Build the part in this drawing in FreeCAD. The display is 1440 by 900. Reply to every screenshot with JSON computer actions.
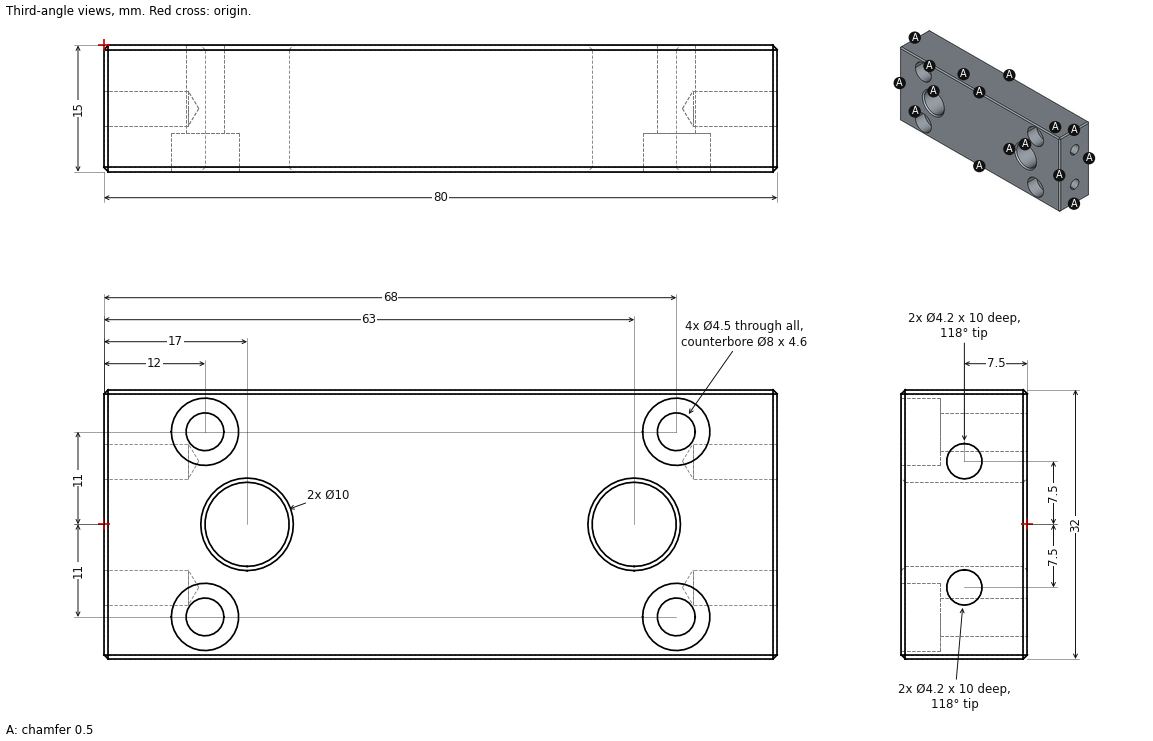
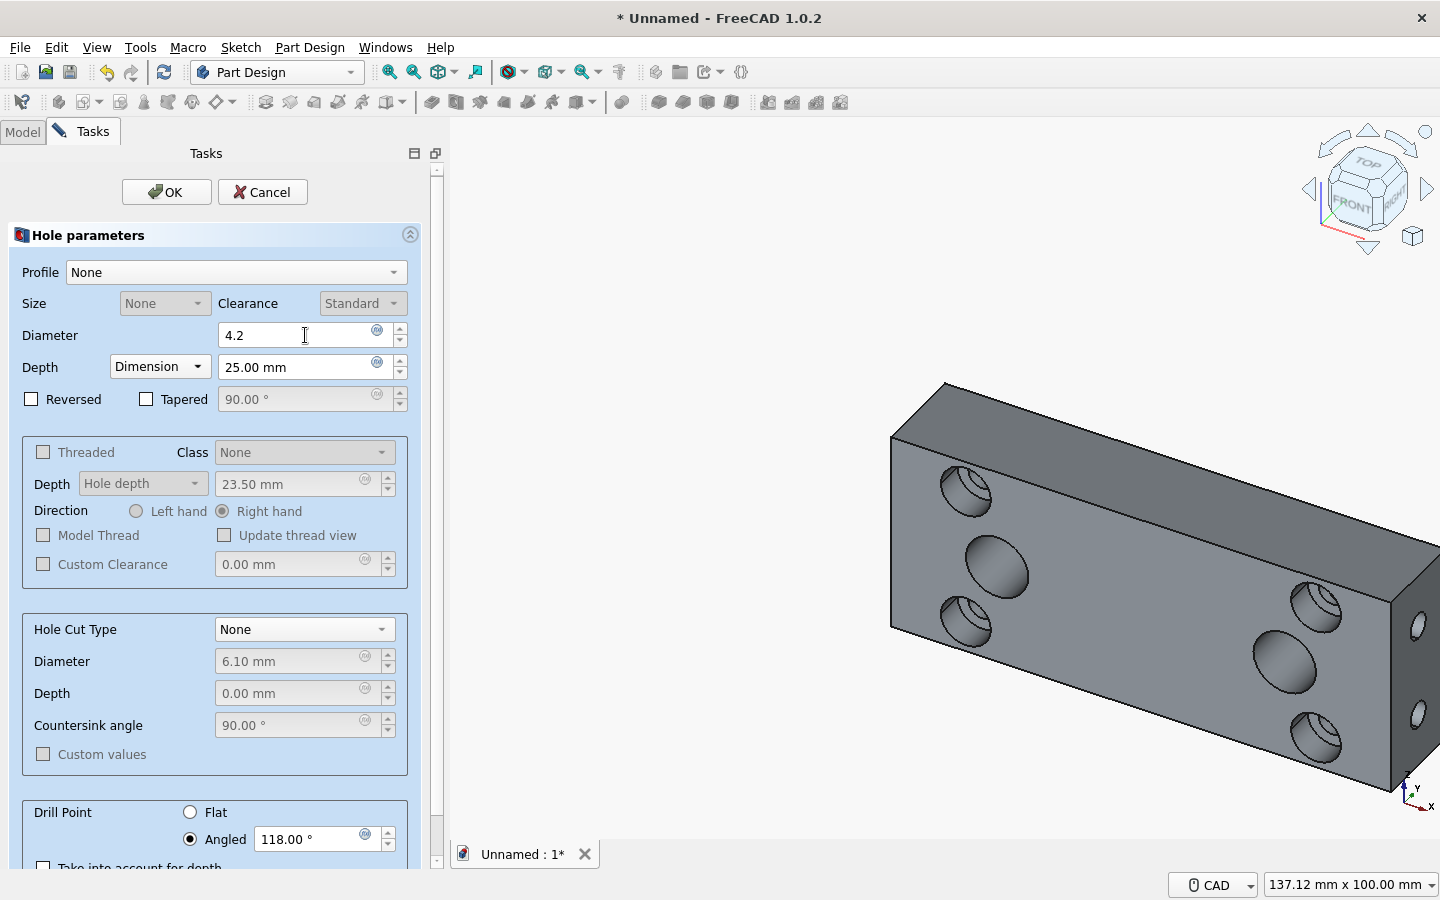
{"action": "triple_click", "coordinate": [305, 367]}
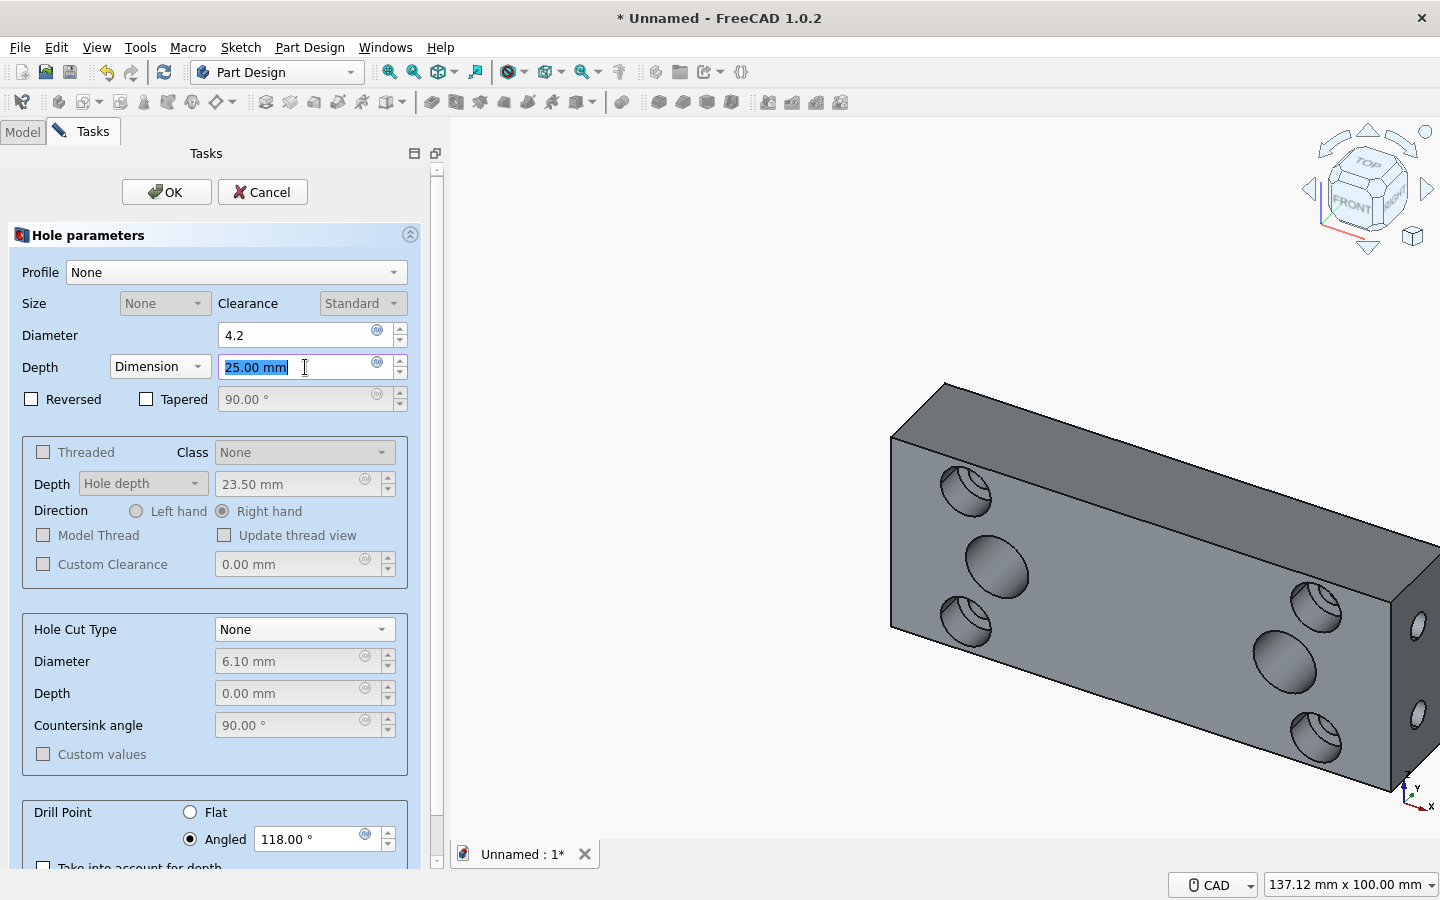
{"action": "type", "text": "10"}
{"action": "key", "text": "Tab"}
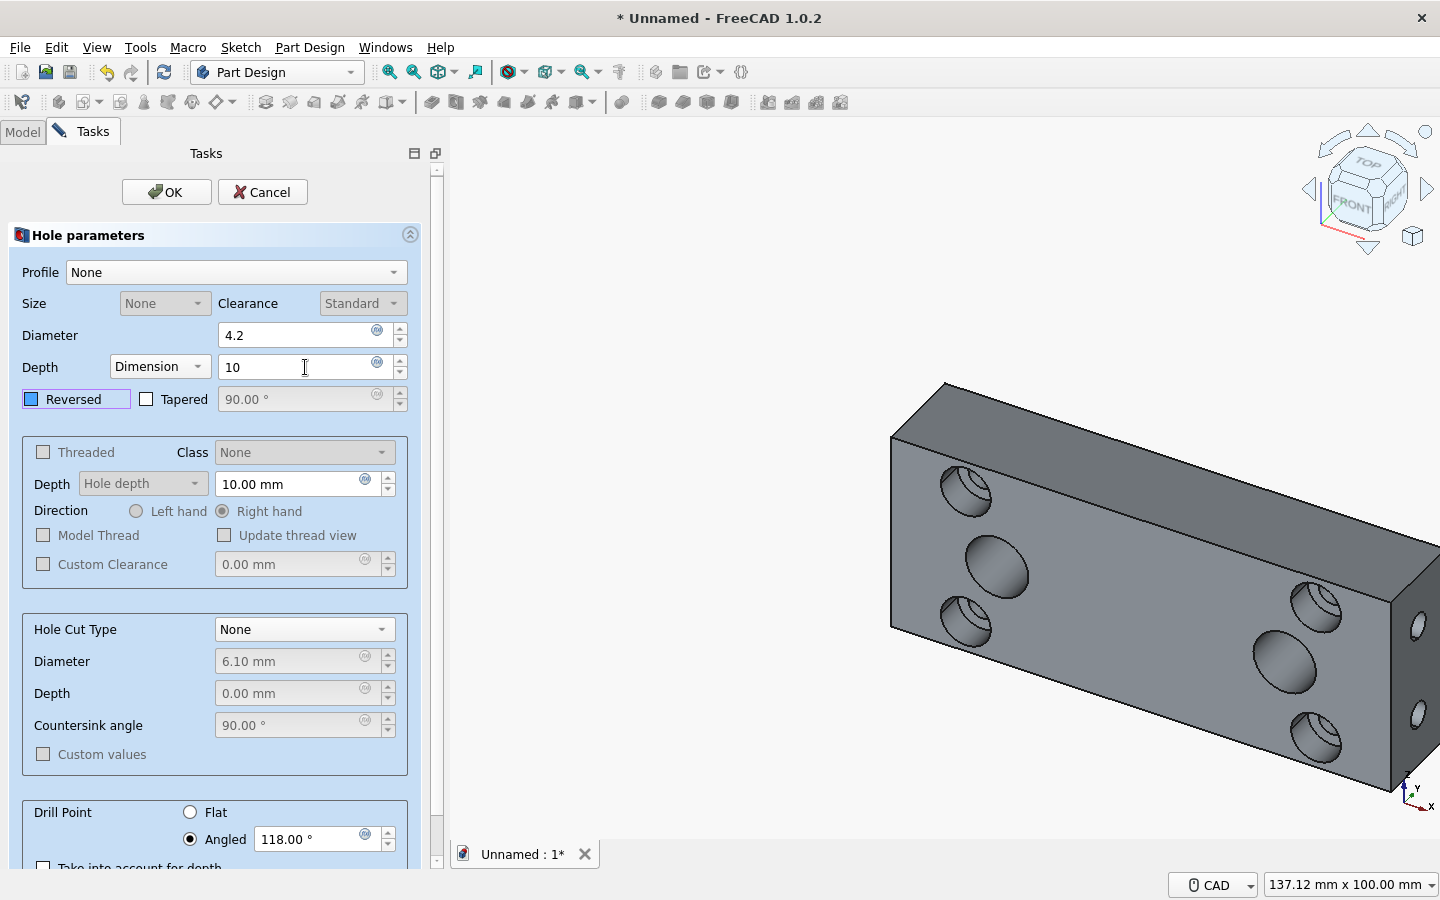
{"action": "left_click", "coordinate": [167, 192]}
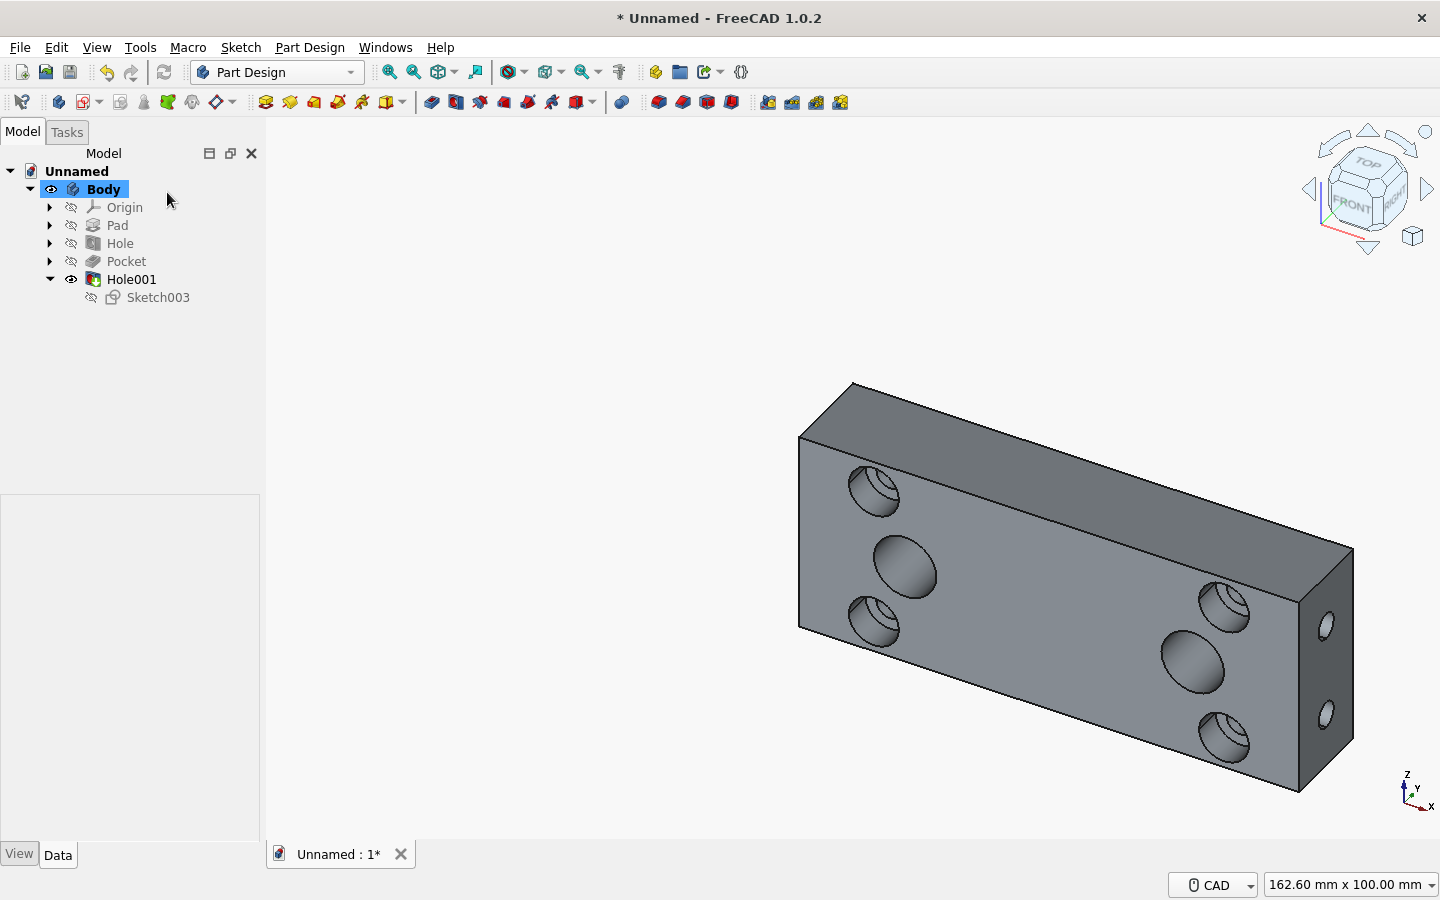
{"action": "key", "text": "6"}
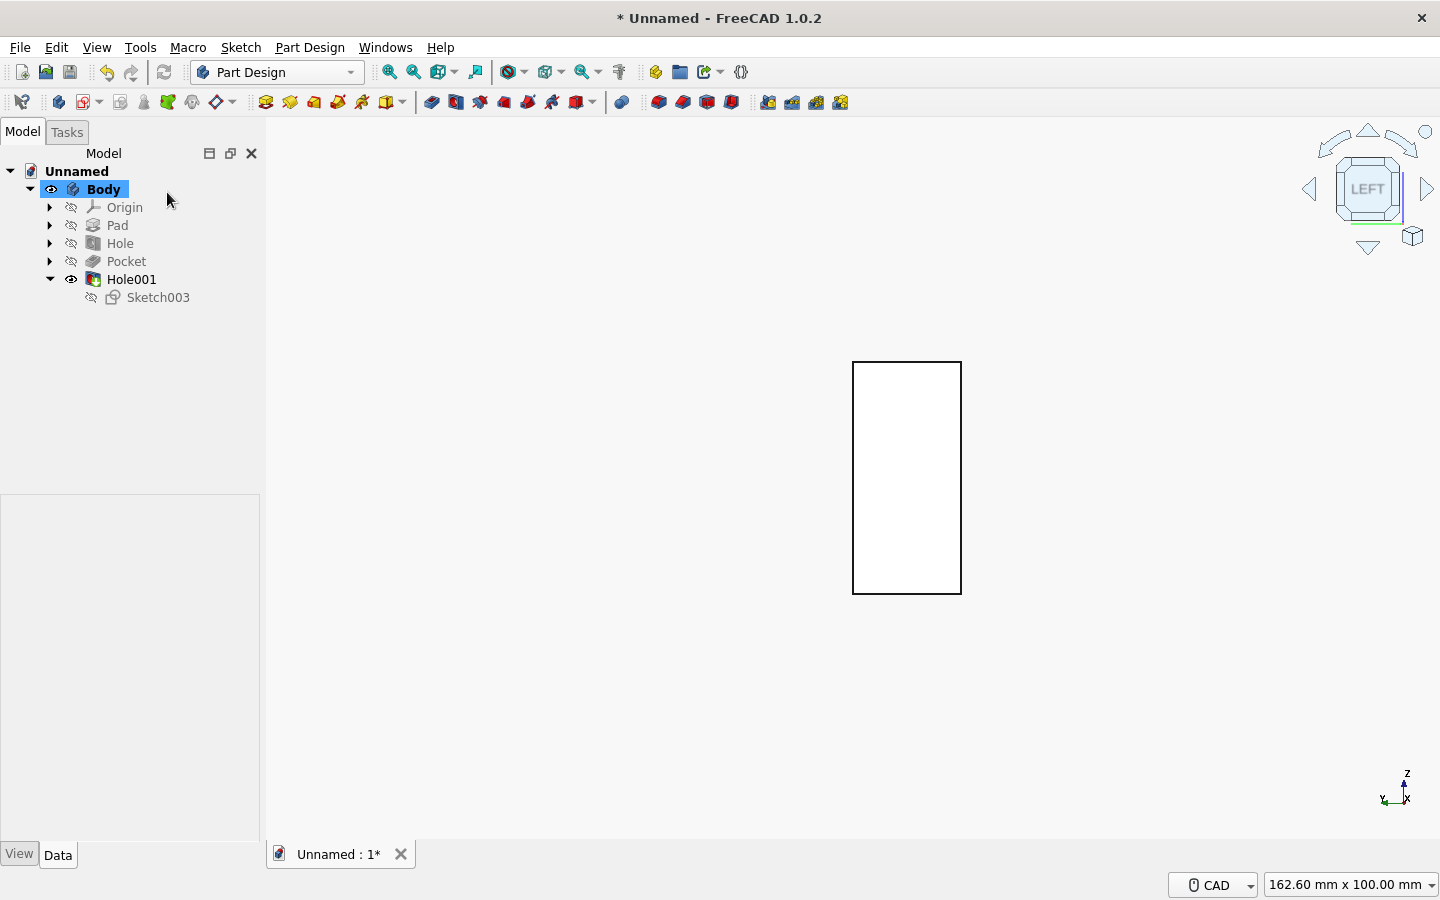
{"action": "left_click", "coordinate": [390, 72]}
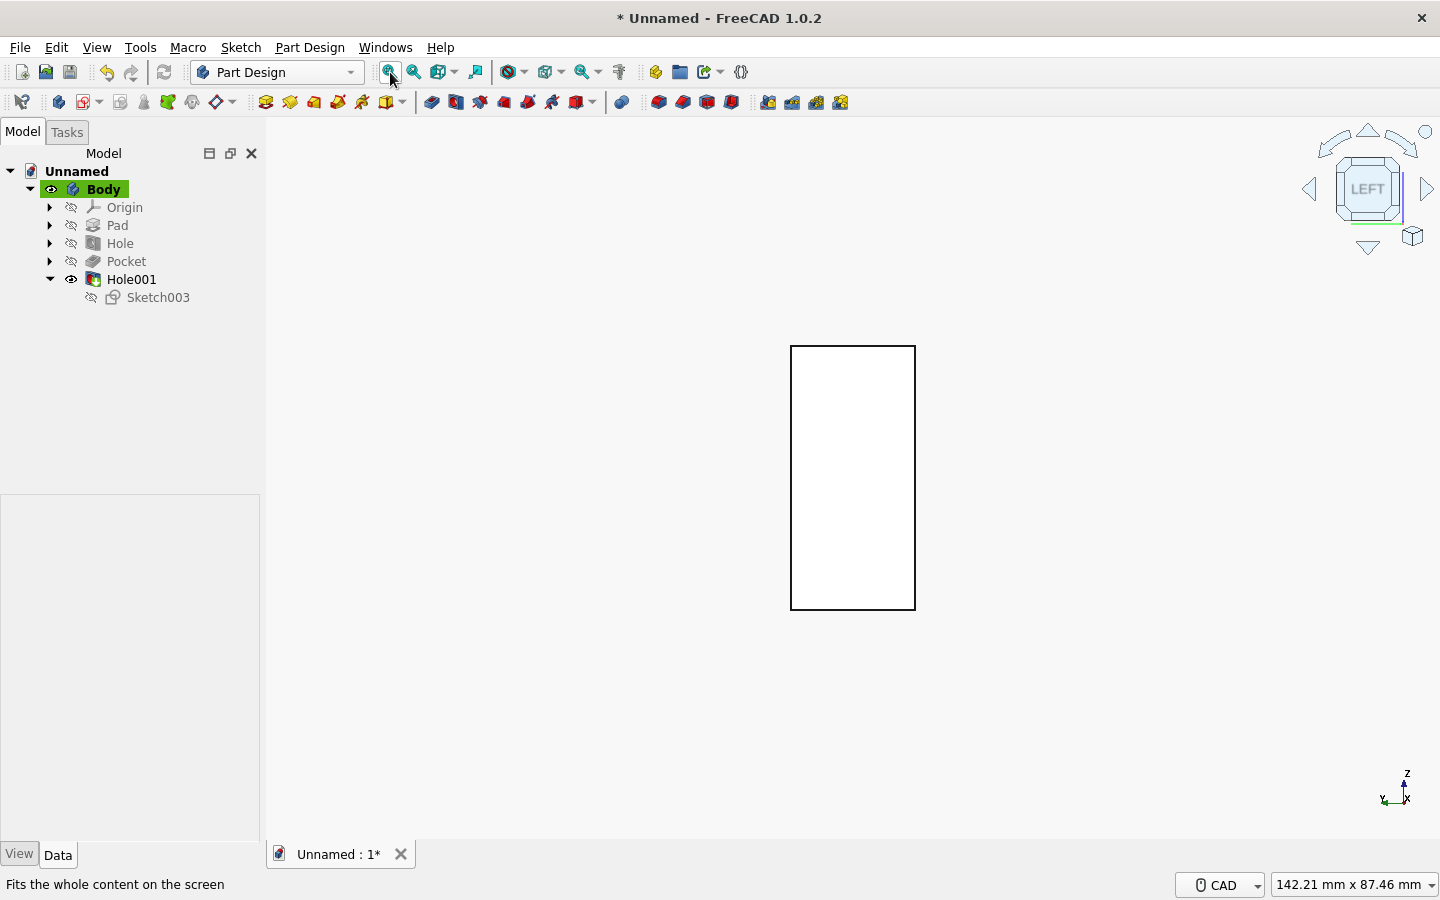
{"action": "left_click", "coordinate": [853, 439]}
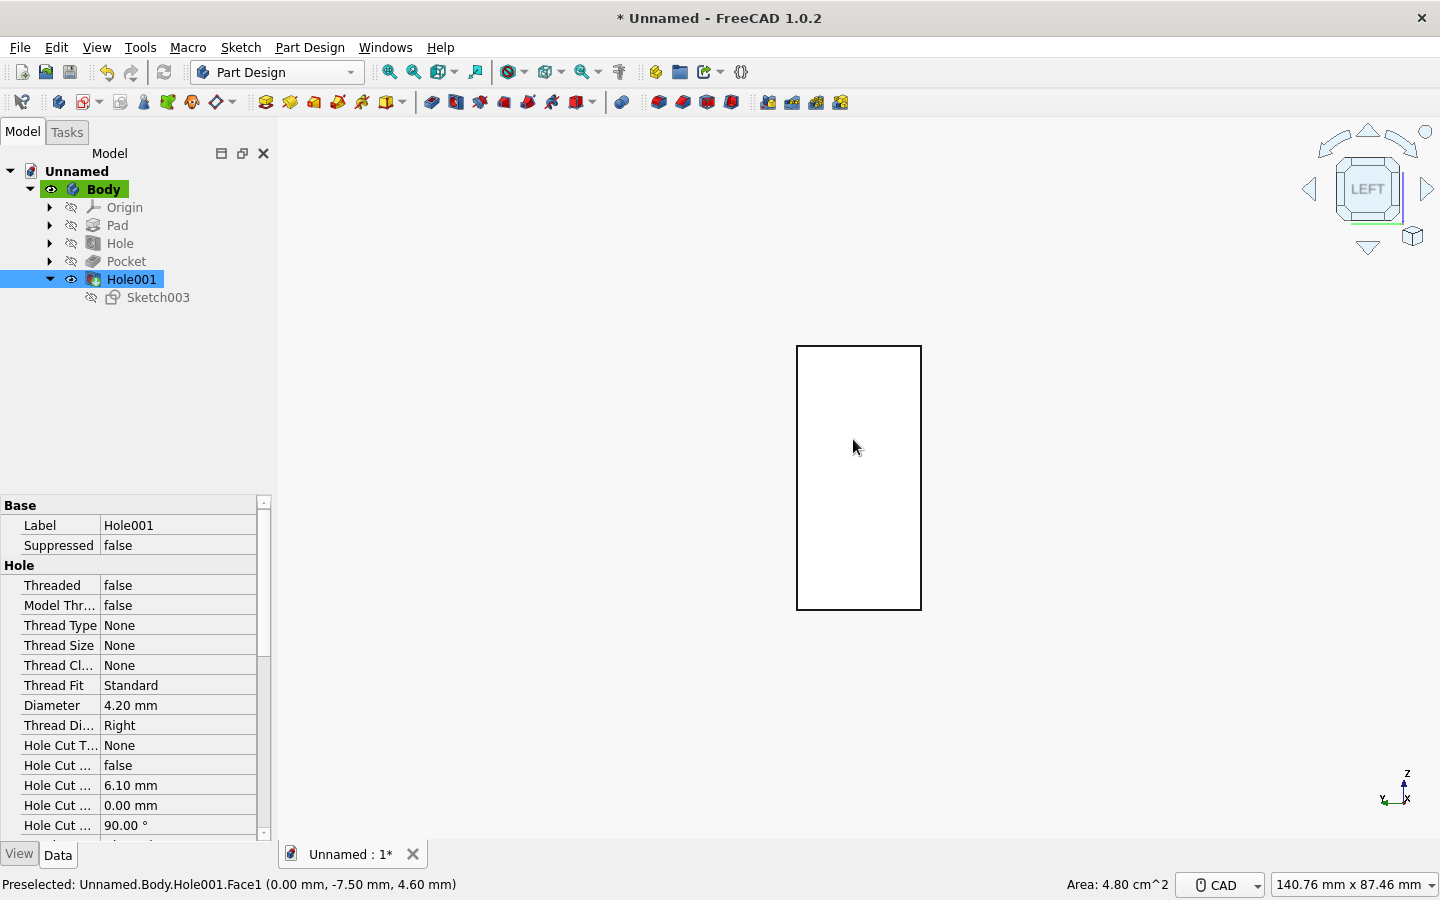
{"action": "left_click", "coordinate": [84, 102]}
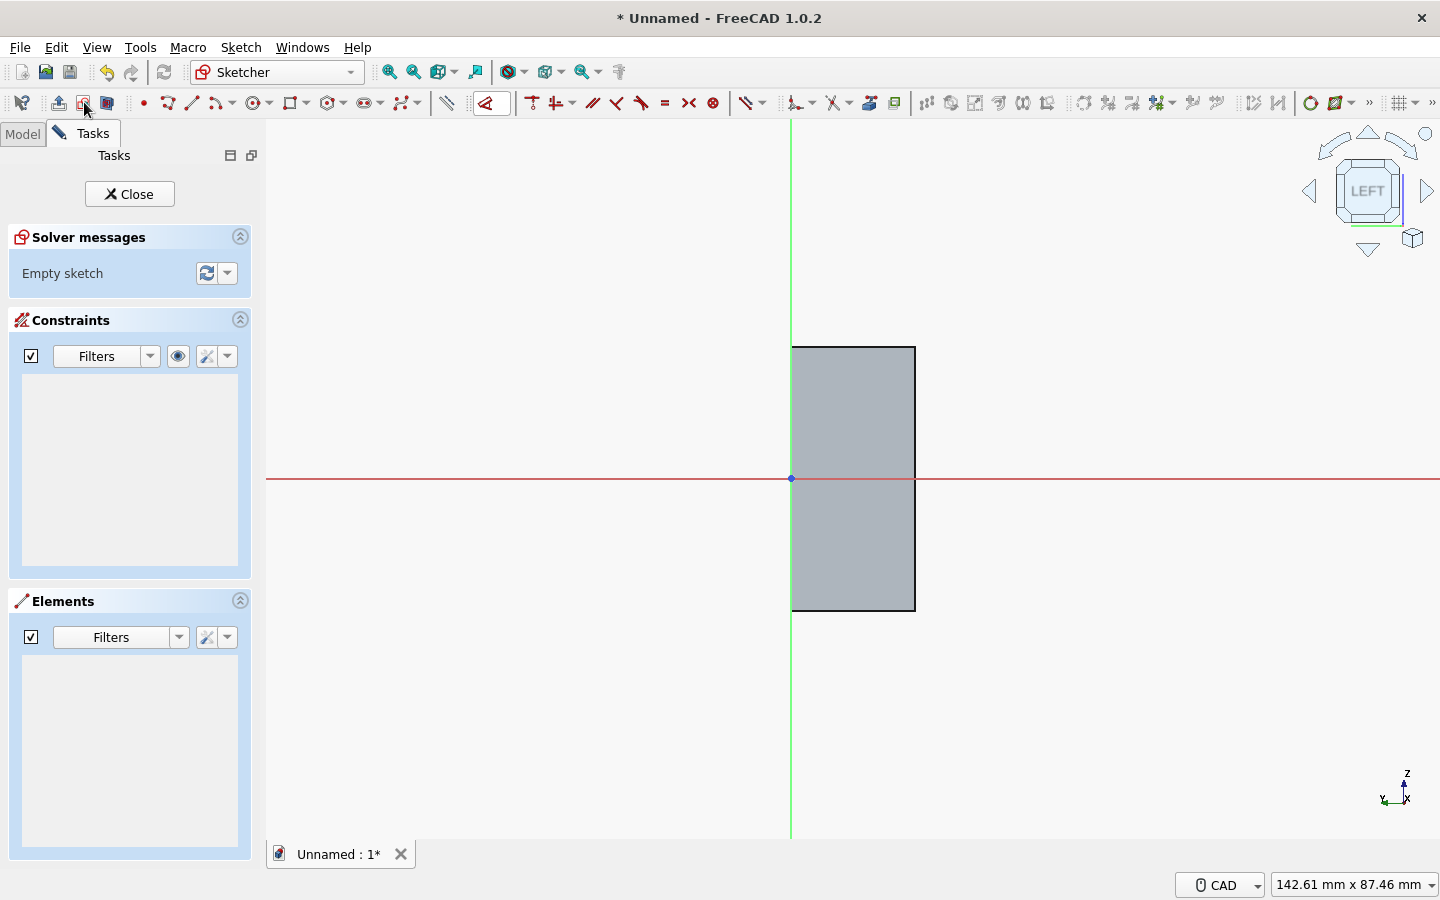
{"action": "scroll", "coordinate": [858, 479], "scroll_direction": "up", "scroll_amount": 5}